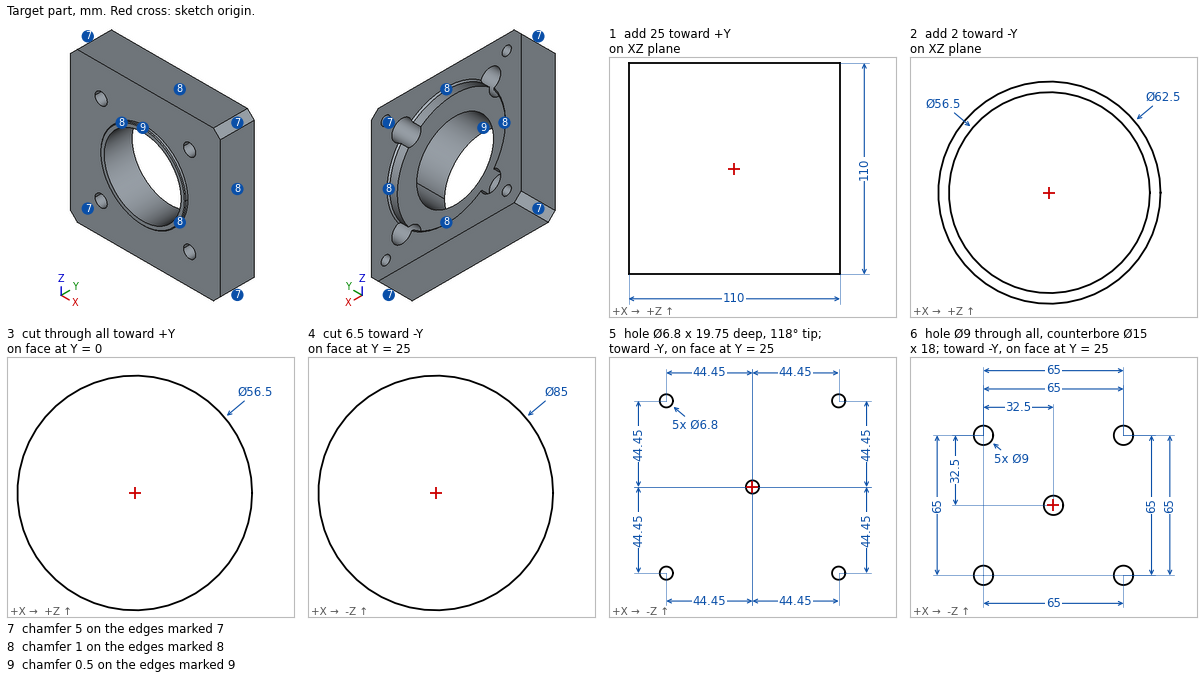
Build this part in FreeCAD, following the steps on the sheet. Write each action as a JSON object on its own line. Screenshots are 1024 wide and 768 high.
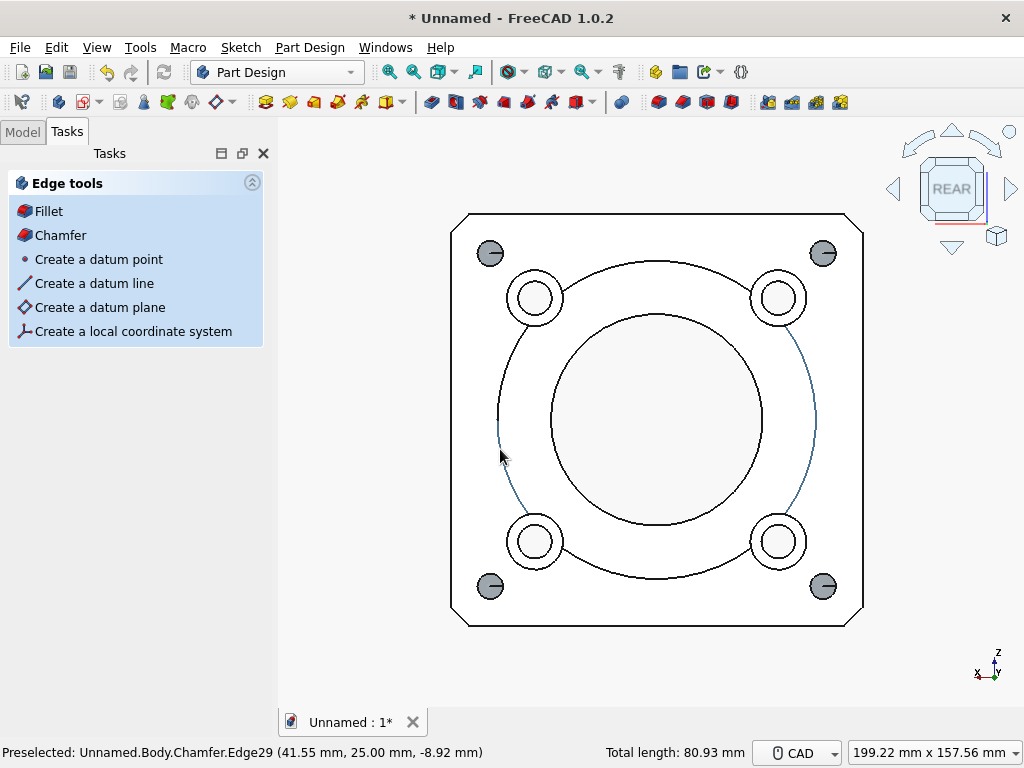
{"action": "left_click", "coordinate": [657, 260], "text": "ctrl"}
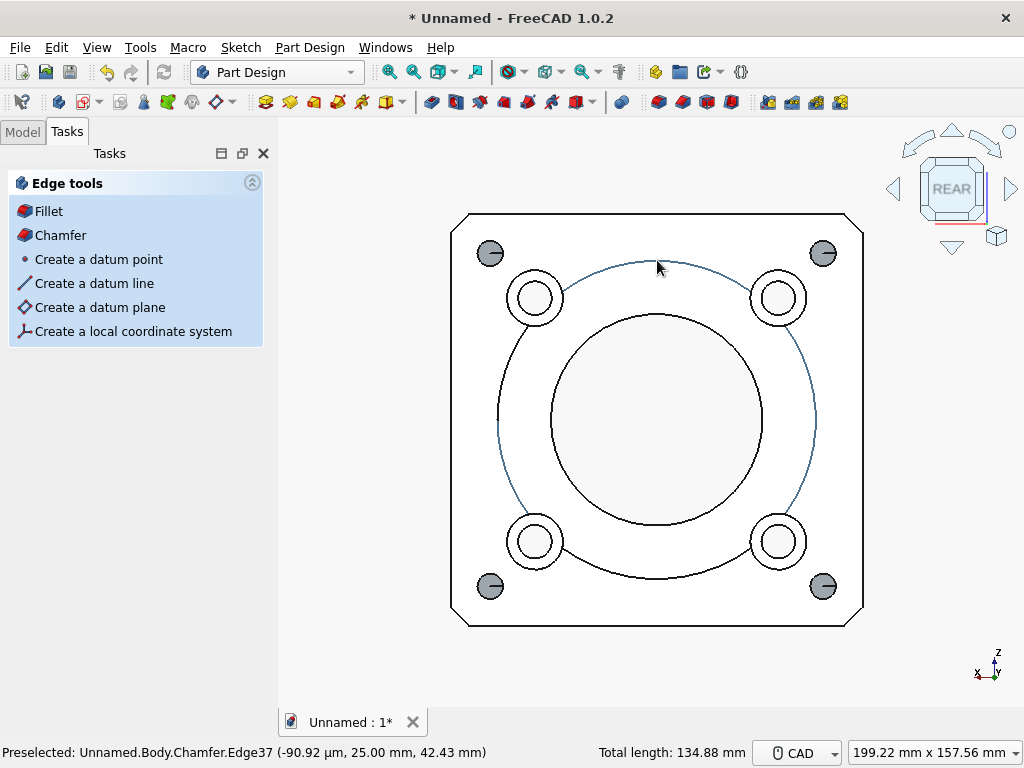
{"action": "key", "text": "6"}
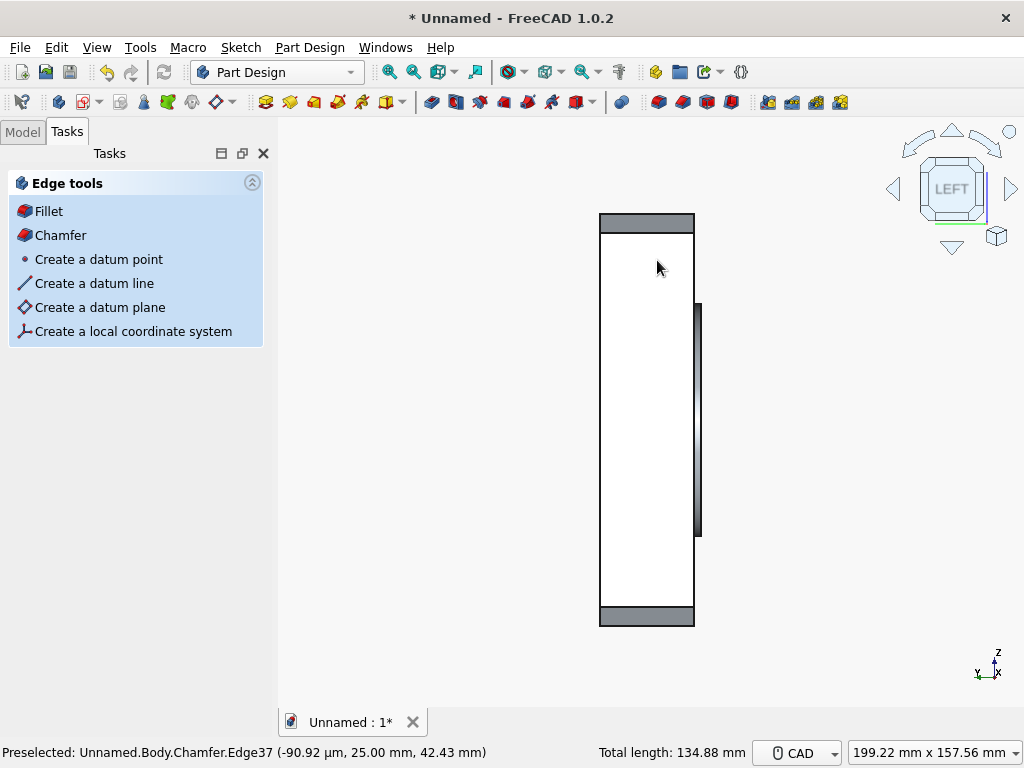
{"action": "key", "text": "v 3"}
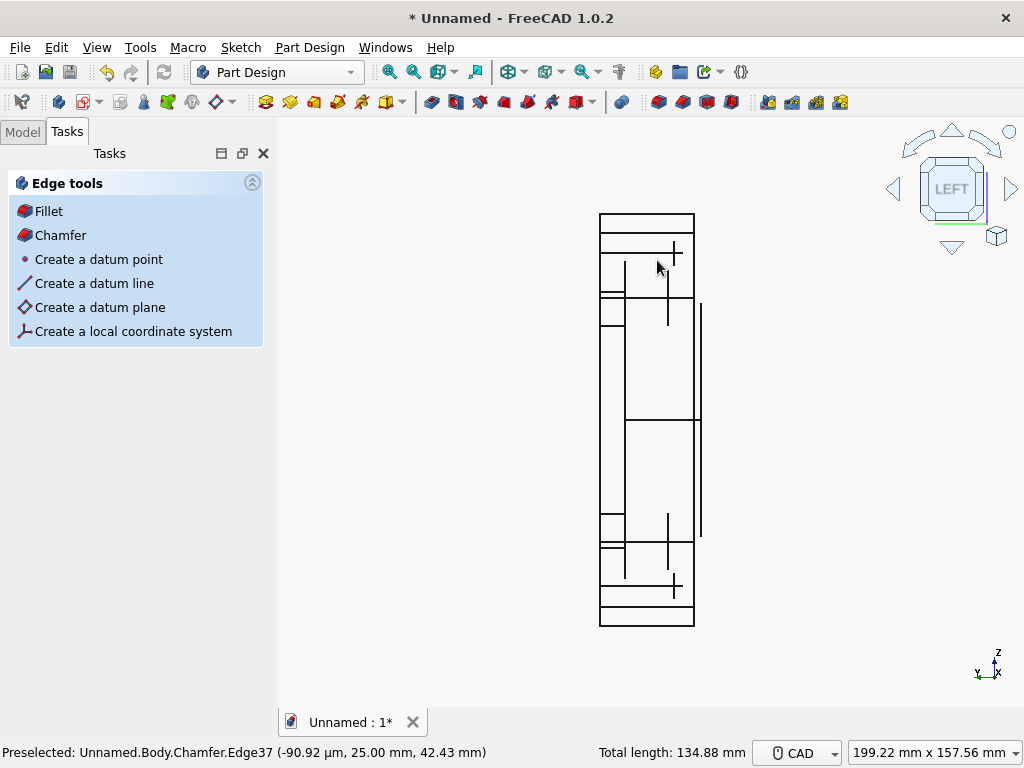
{"action": "key", "text": "0"}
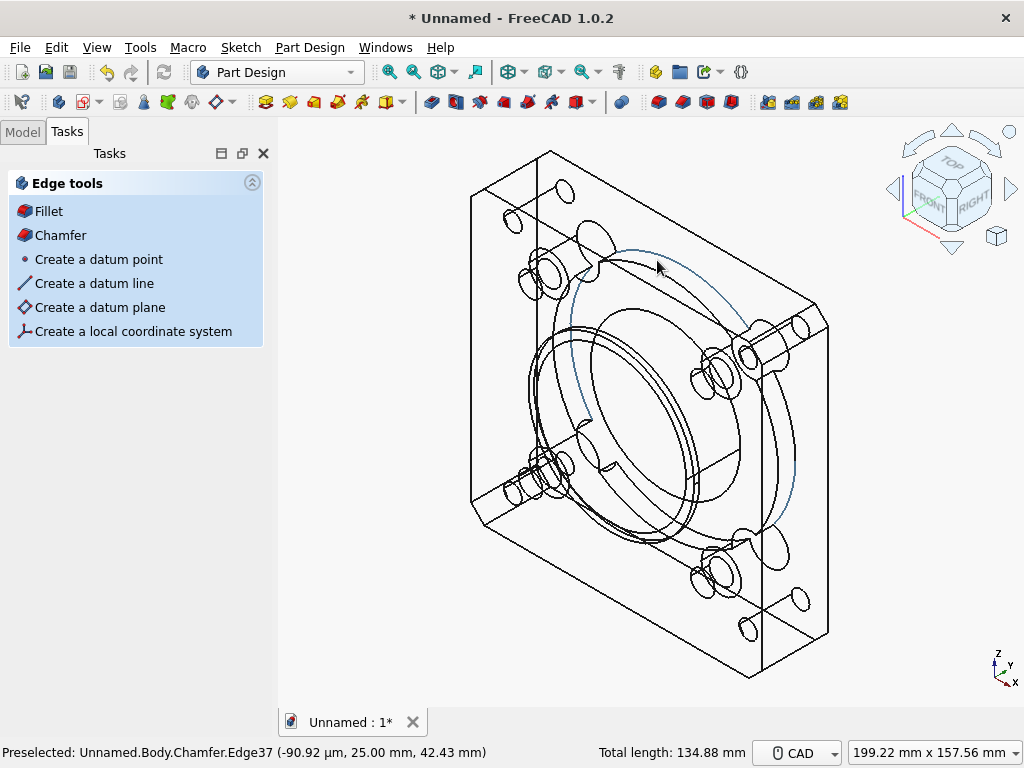
{"action": "left_click", "coordinate": [697, 532], "text": "ctrl"}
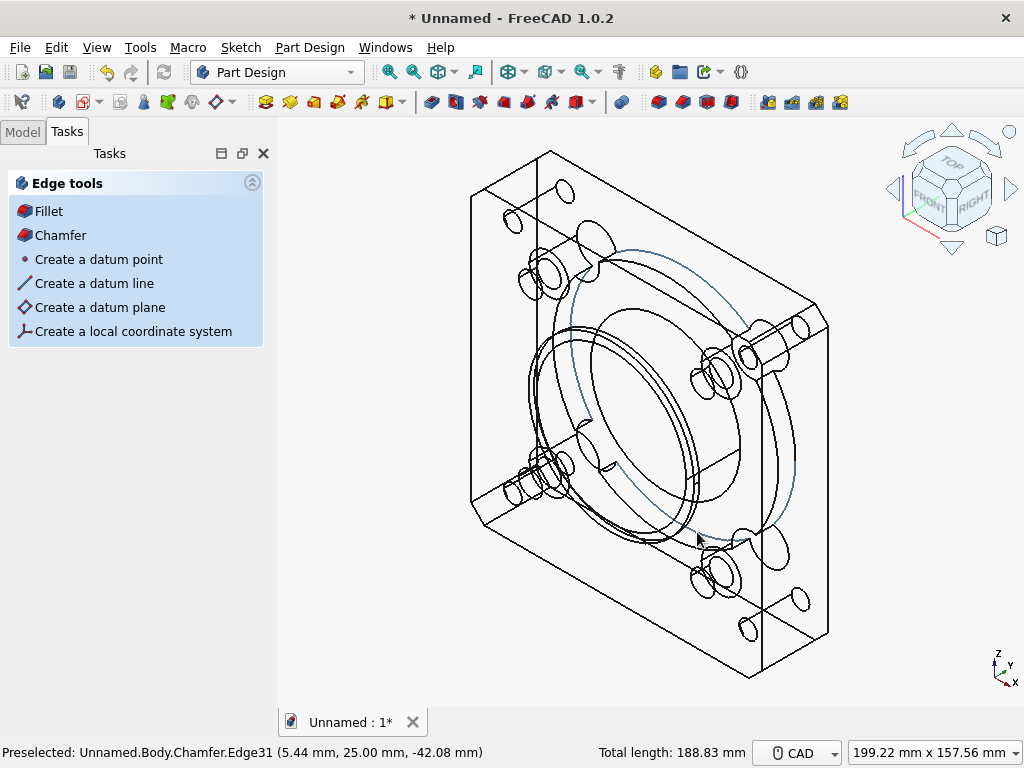
{"action": "key", "text": "v 1"}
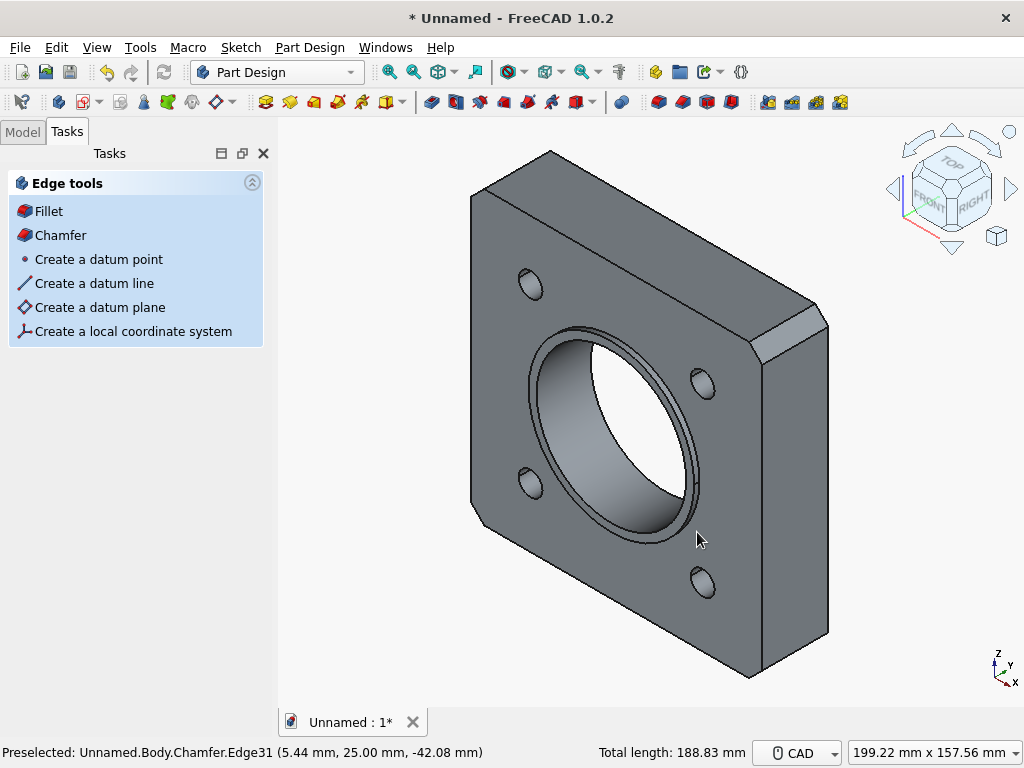
{"action": "left_click", "coordinate": [684, 102]}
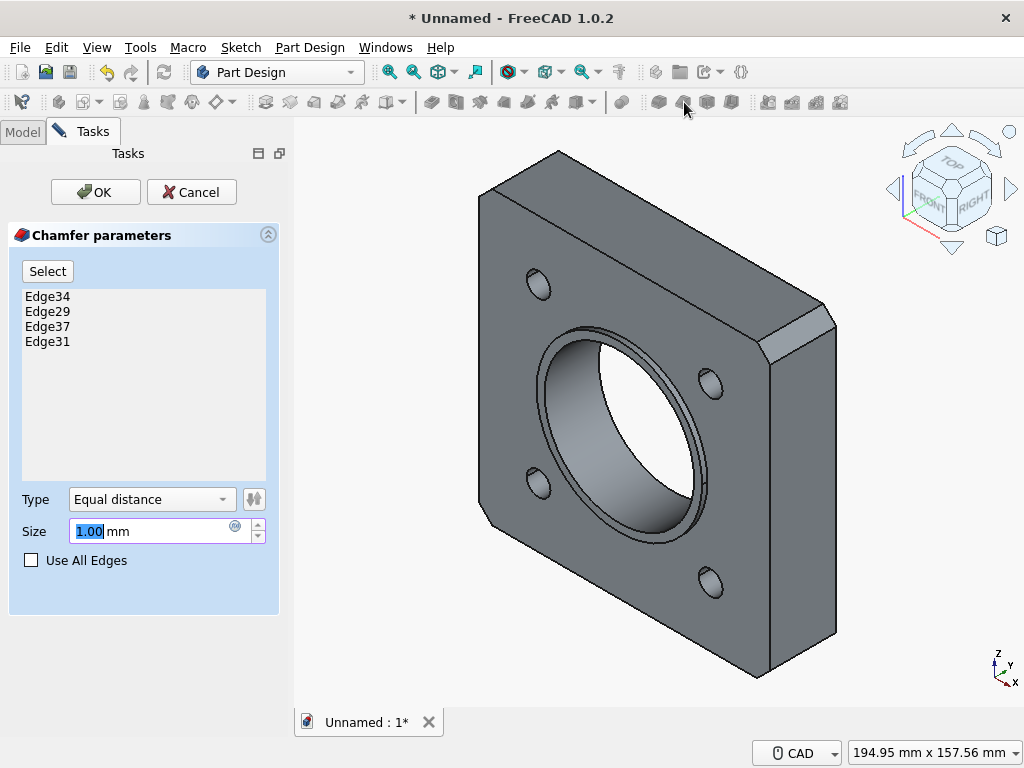
{"action": "type", "text": "1"}
{"action": "key", "text": "Tab"}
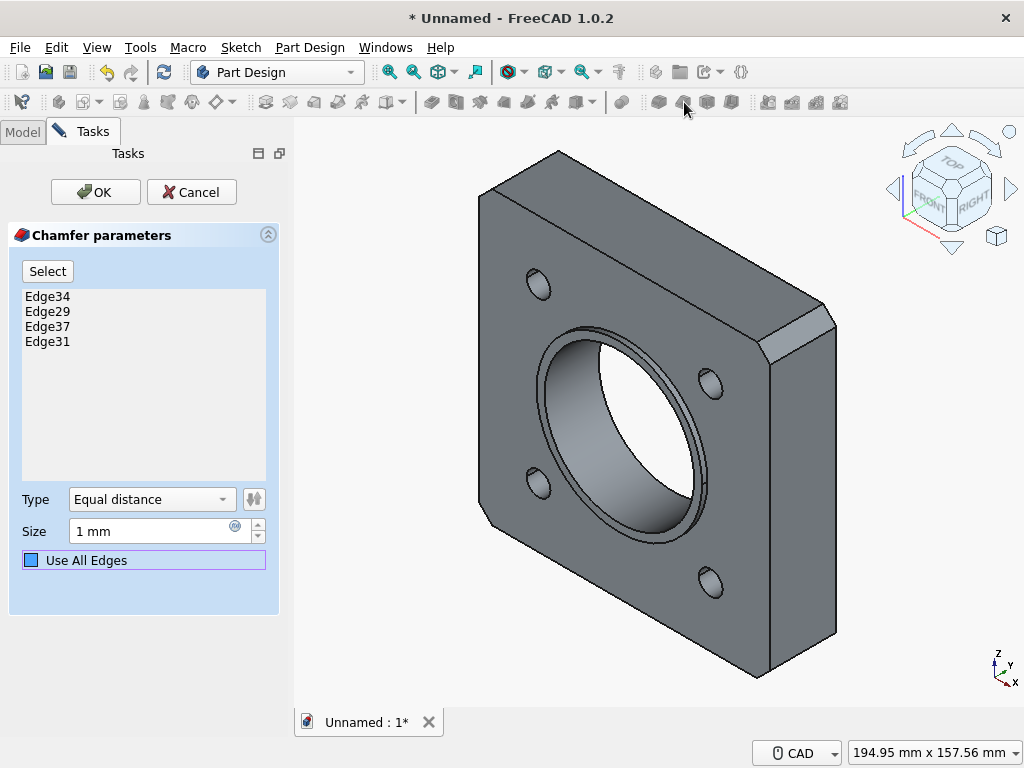
{"action": "left_click", "coordinate": [96, 192]}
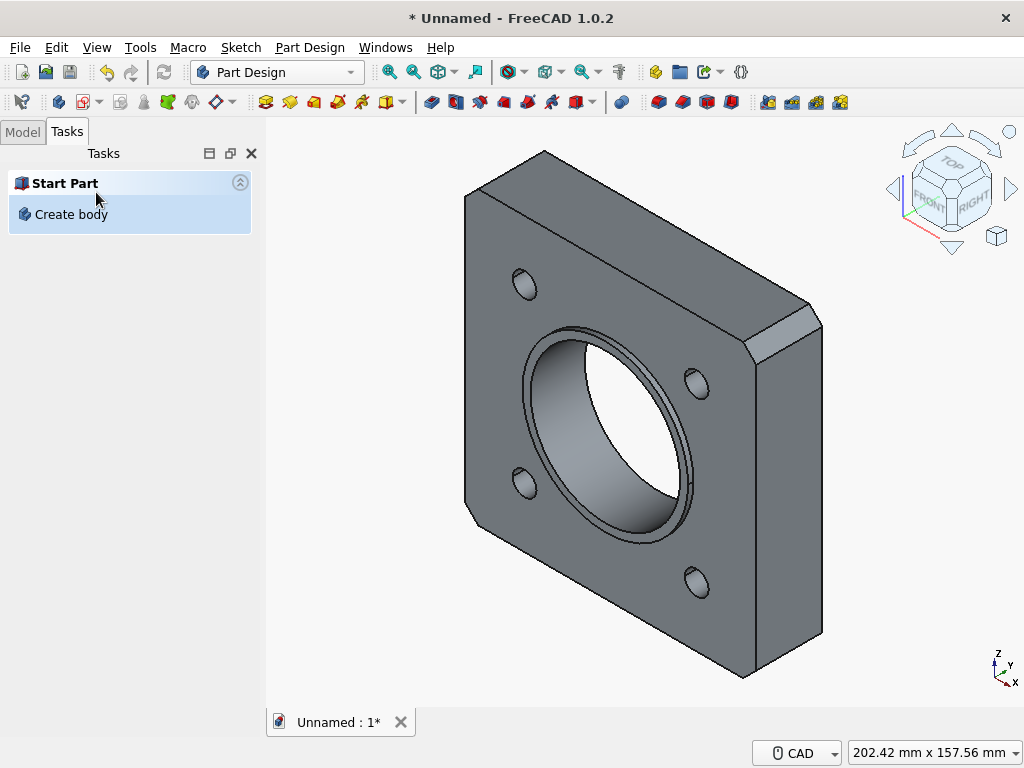
{"action": "left_click", "coordinate": [580, 330]}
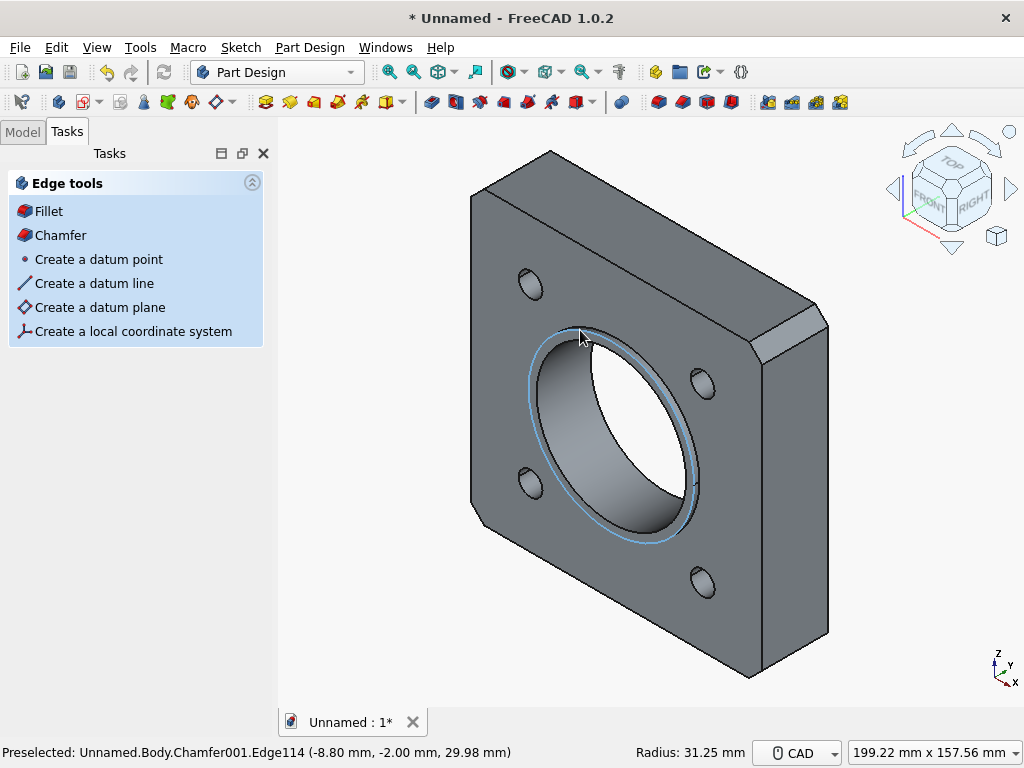
{"action": "left_click", "coordinate": [684, 102]}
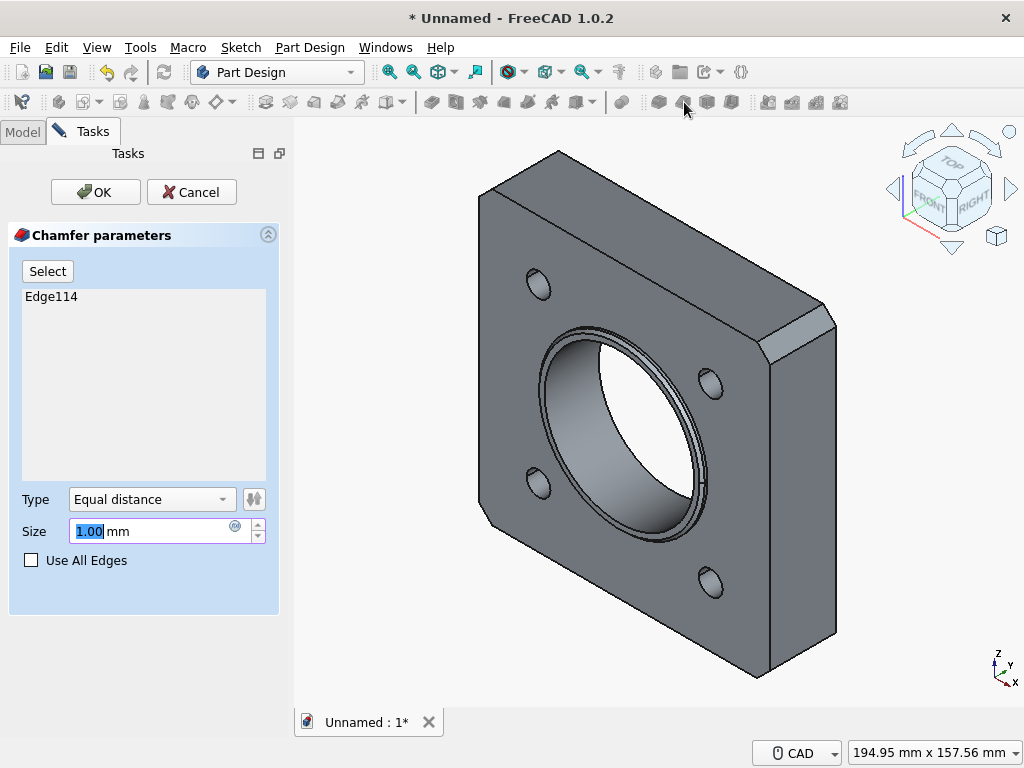
{"action": "type", "text": "0.5"}
{"action": "key", "text": "Tab"}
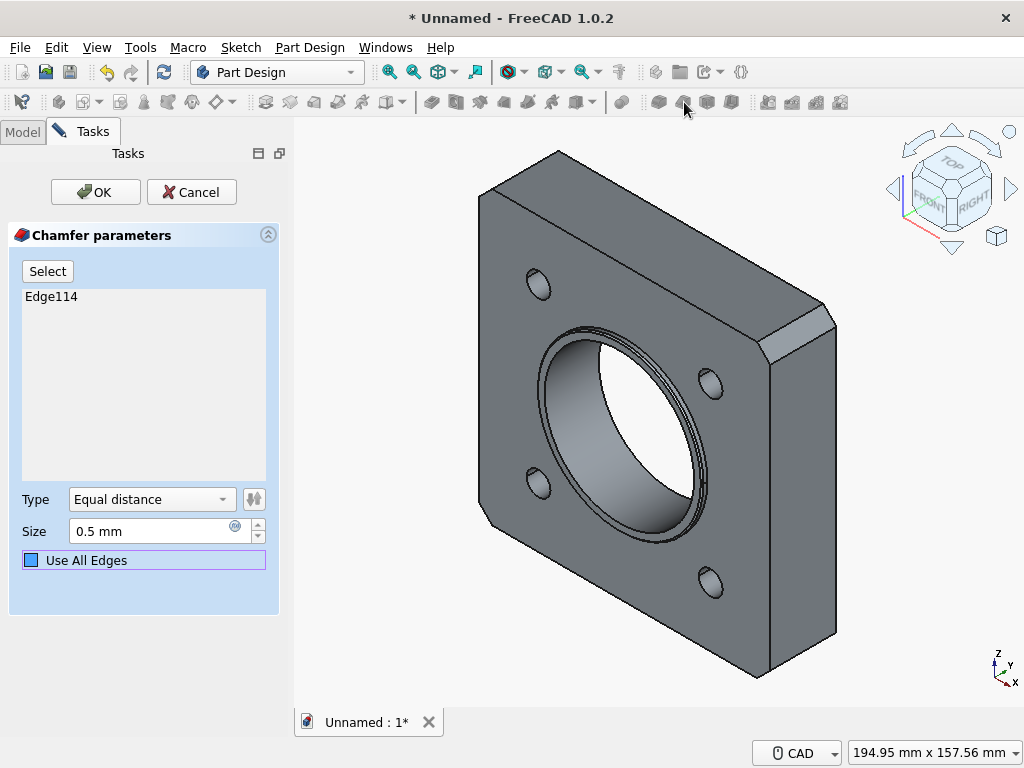
{"action": "left_click", "coordinate": [96, 192]}